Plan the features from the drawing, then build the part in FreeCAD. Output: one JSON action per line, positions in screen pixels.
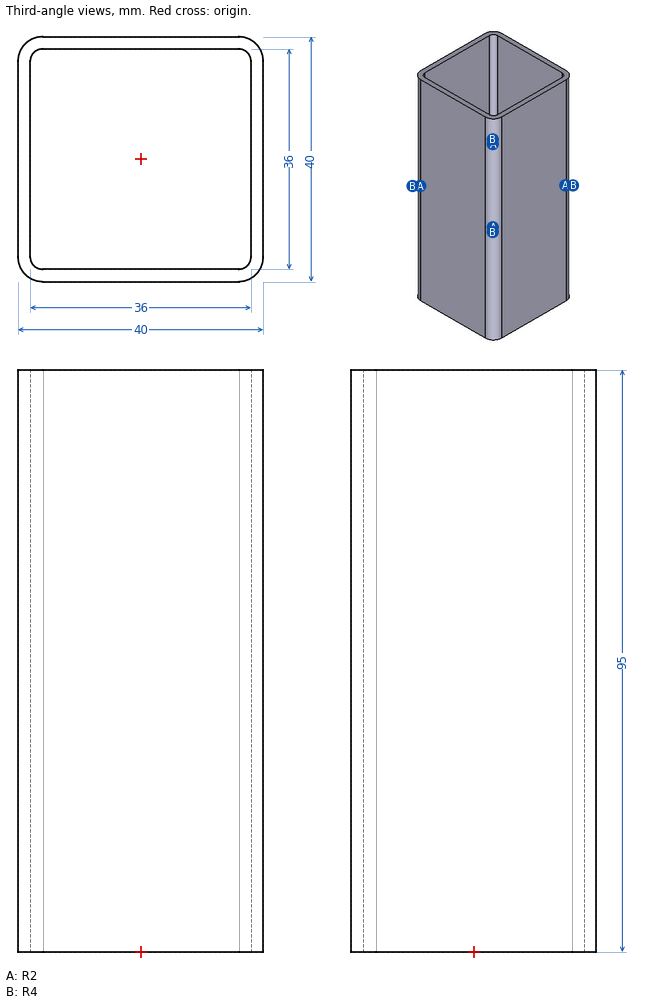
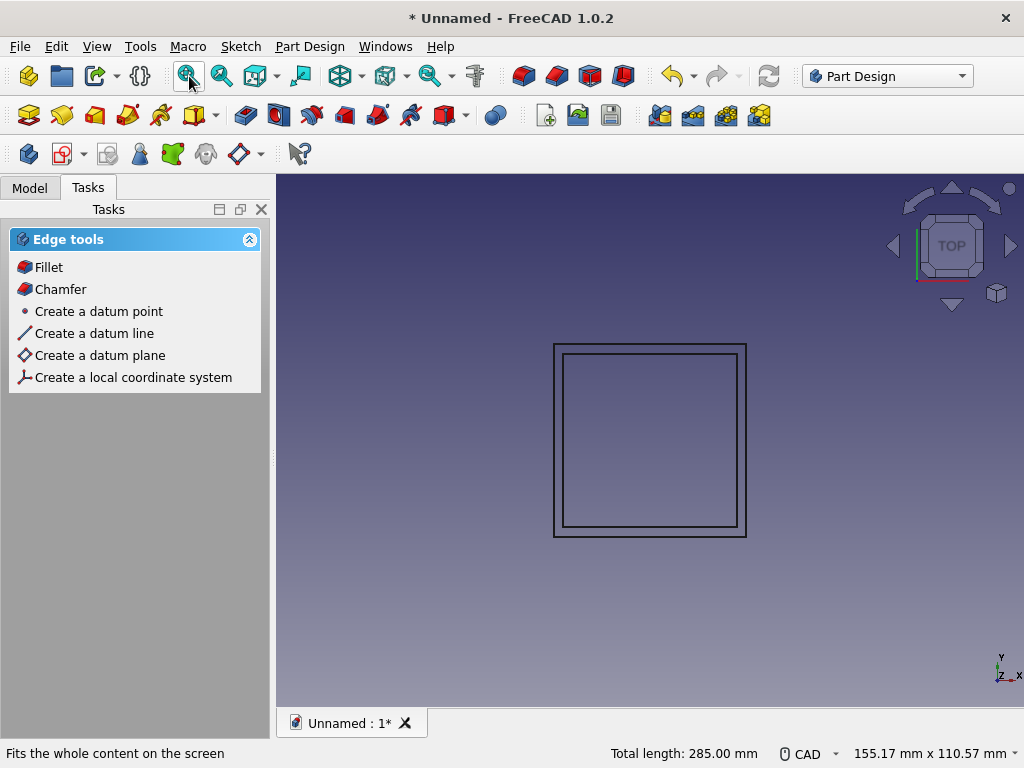
{"action": "key", "text": "v f"}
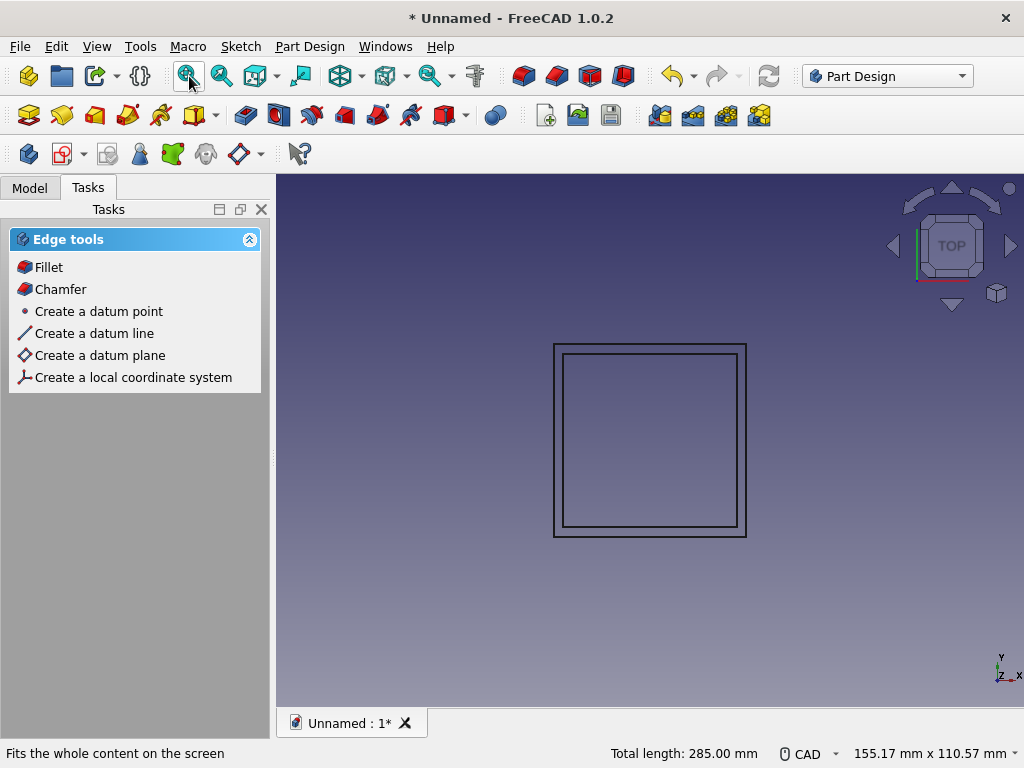
{"action": "scroll", "coordinate": [737, 526], "scroll_direction": "up", "scroll_amount": 6}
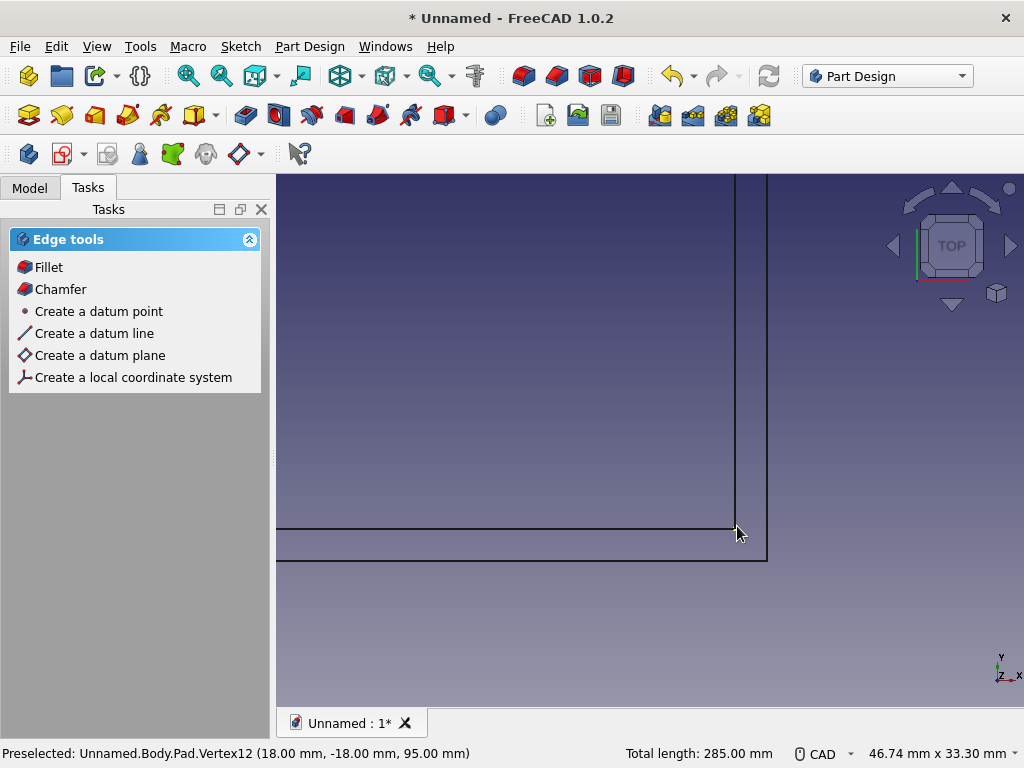
{"action": "key", "text": "v f"}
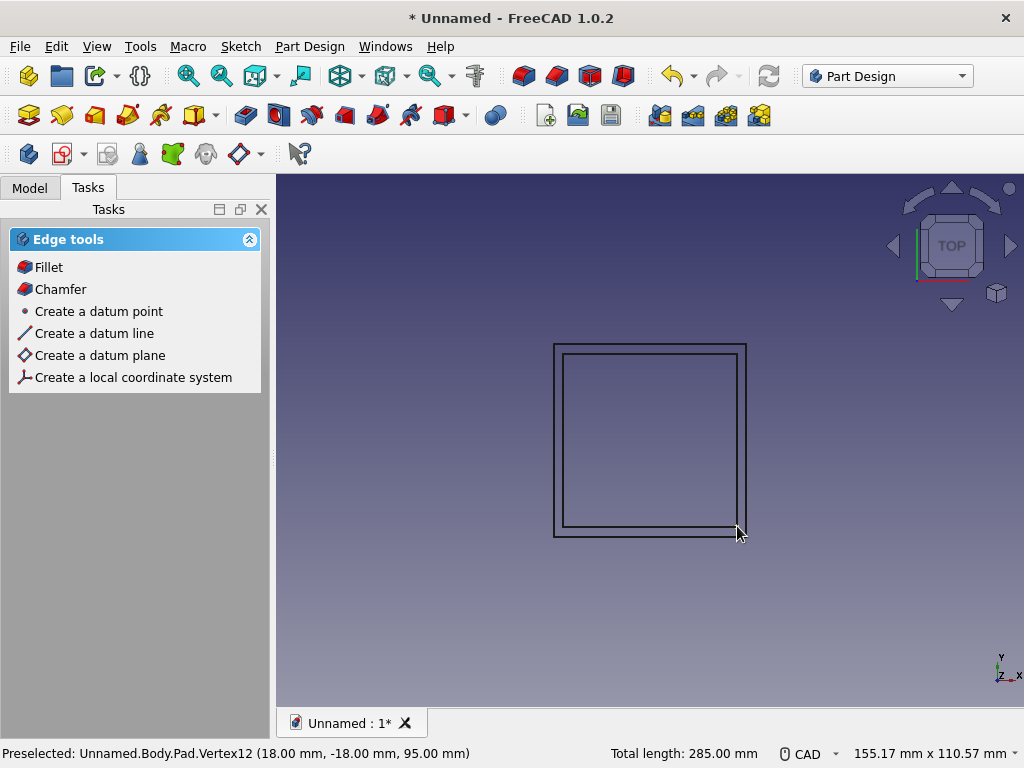
{"action": "key", "text": "1"}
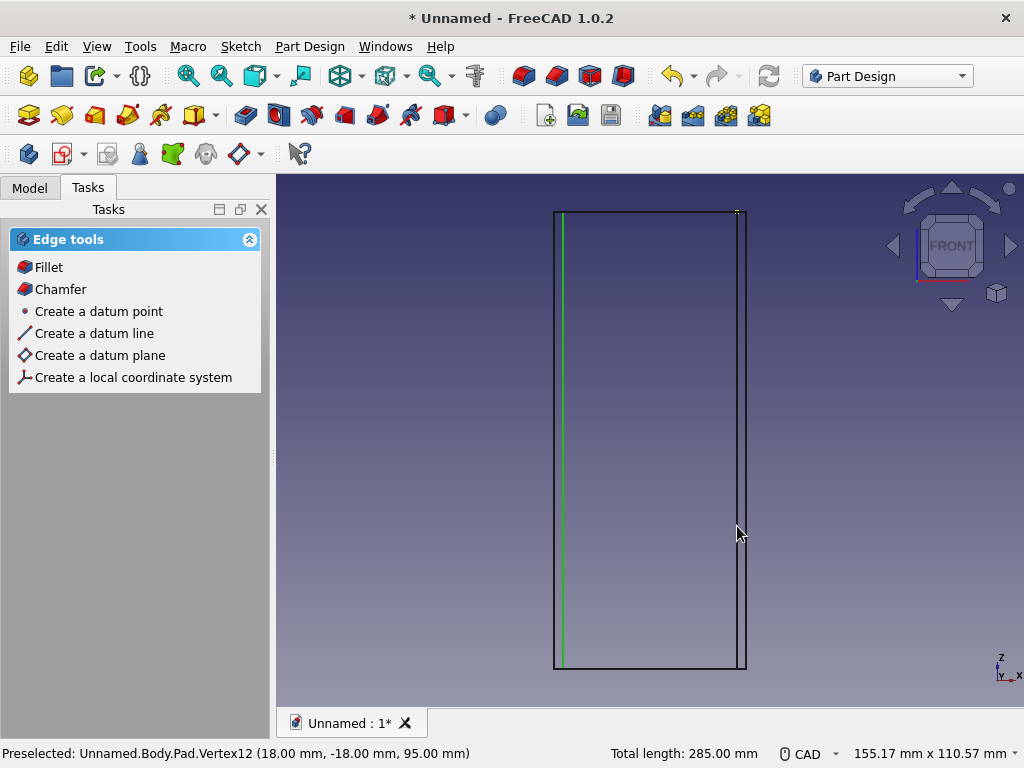
{"action": "left_click", "coordinate": [737, 439], "text": "ctrl"}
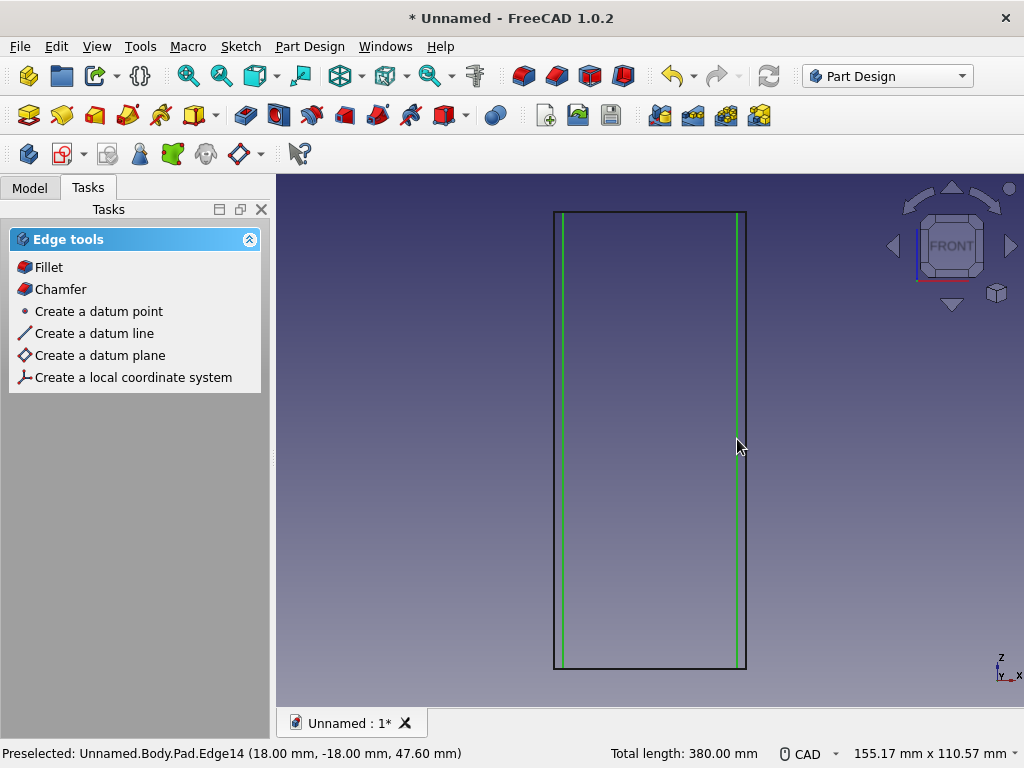
{"action": "key", "text": "v 1"}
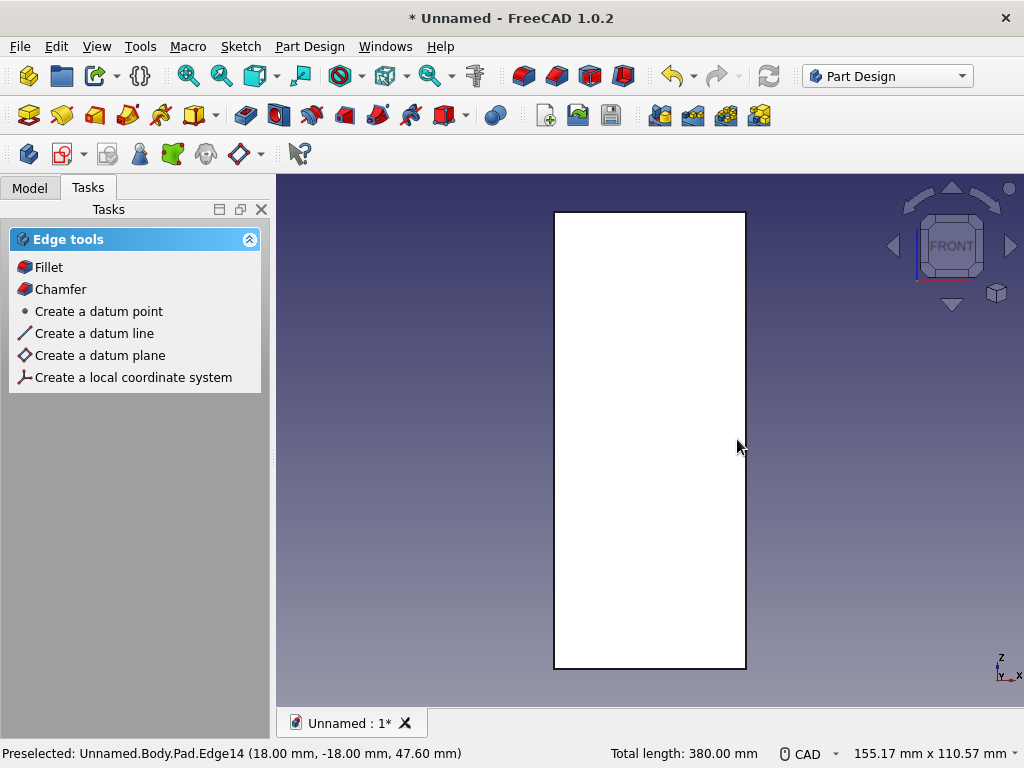
{"action": "left_click", "coordinate": [524, 76]}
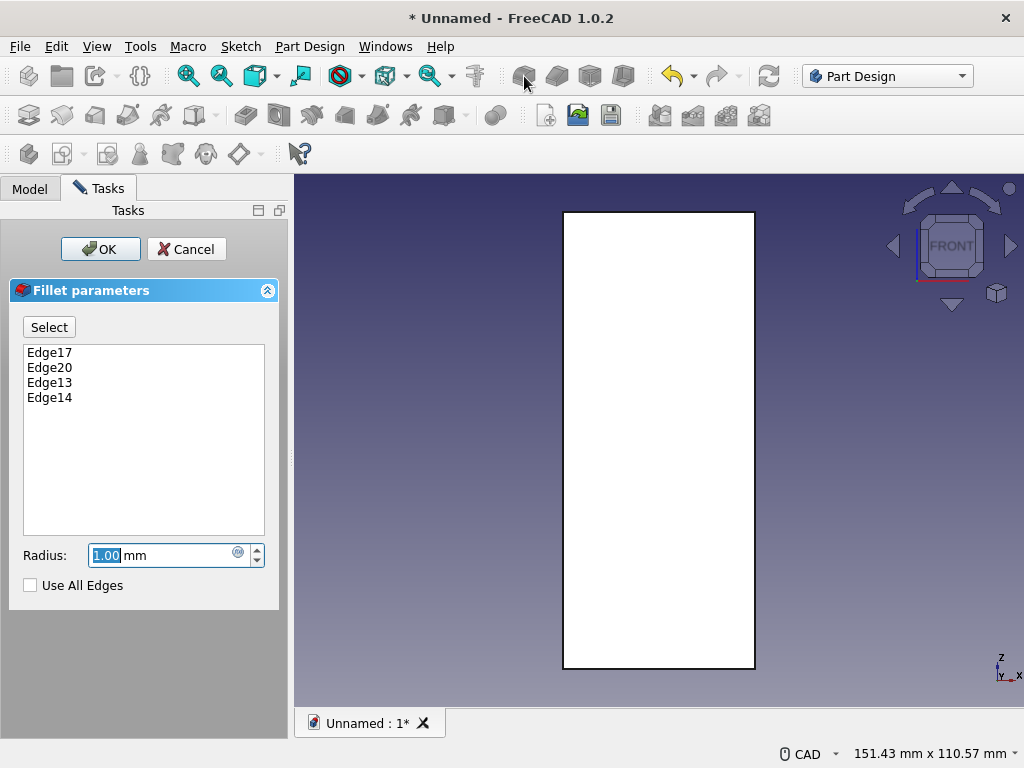
{"action": "type", "text": "2"}
{"action": "key", "text": "Tab"}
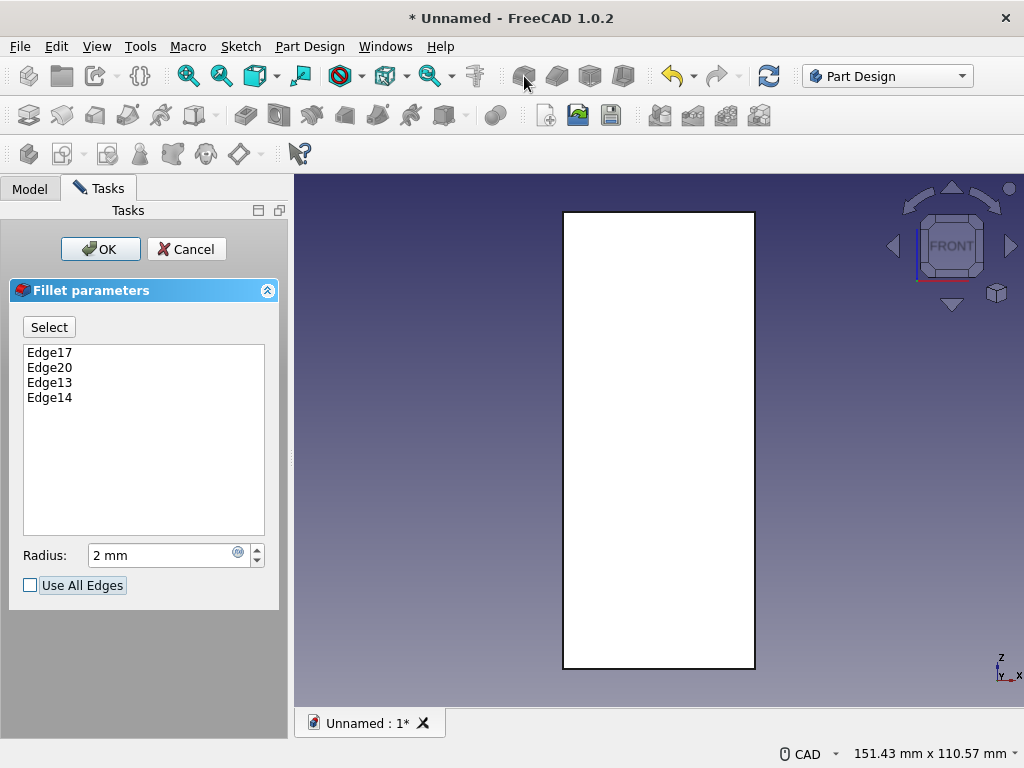
{"action": "left_click", "coordinate": [101, 249]}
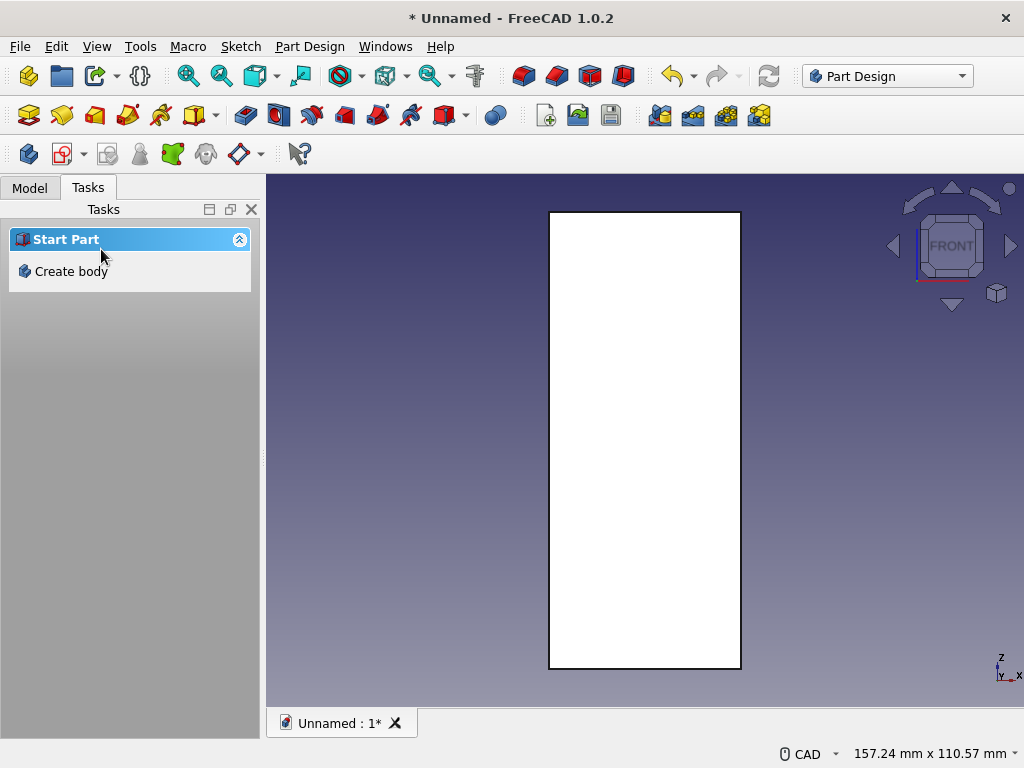
{"action": "left_click", "coordinate": [741, 439]}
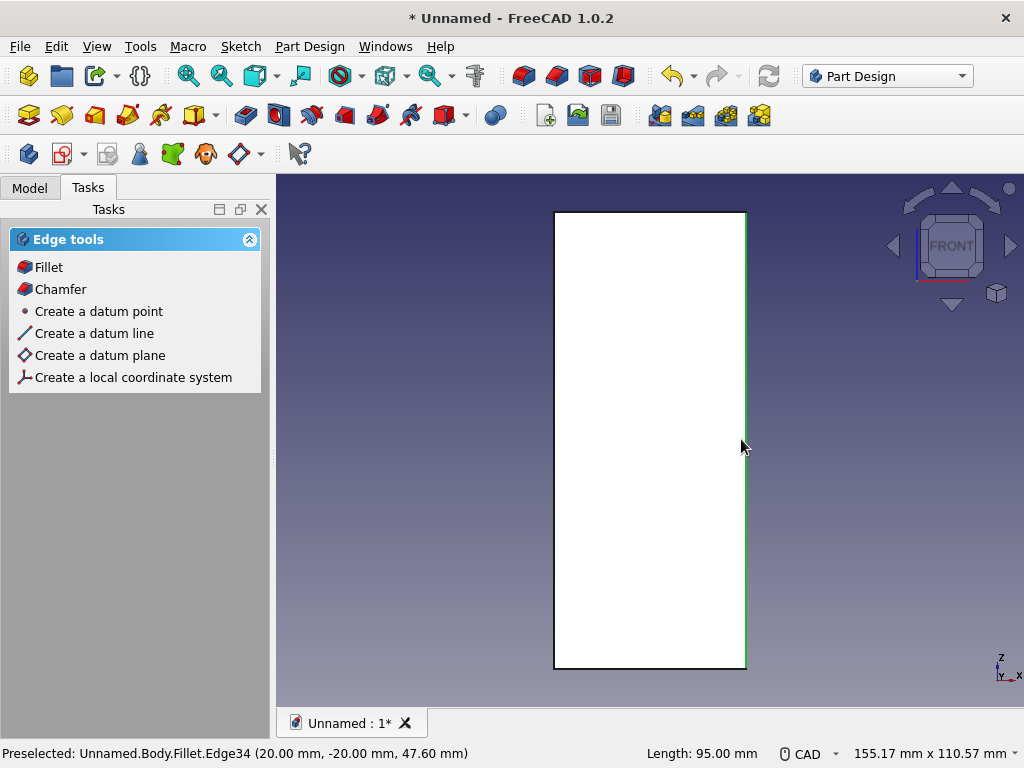
{"action": "left_click", "coordinate": [554, 439], "text": "ctrl"}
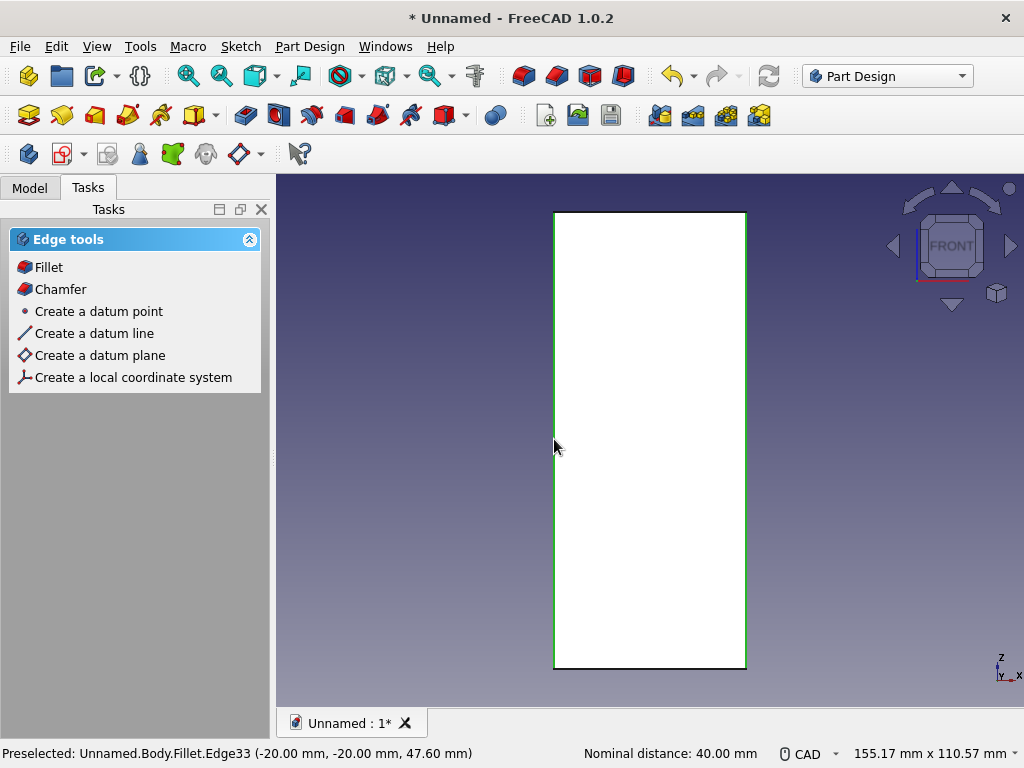
{"action": "key", "text": "0"}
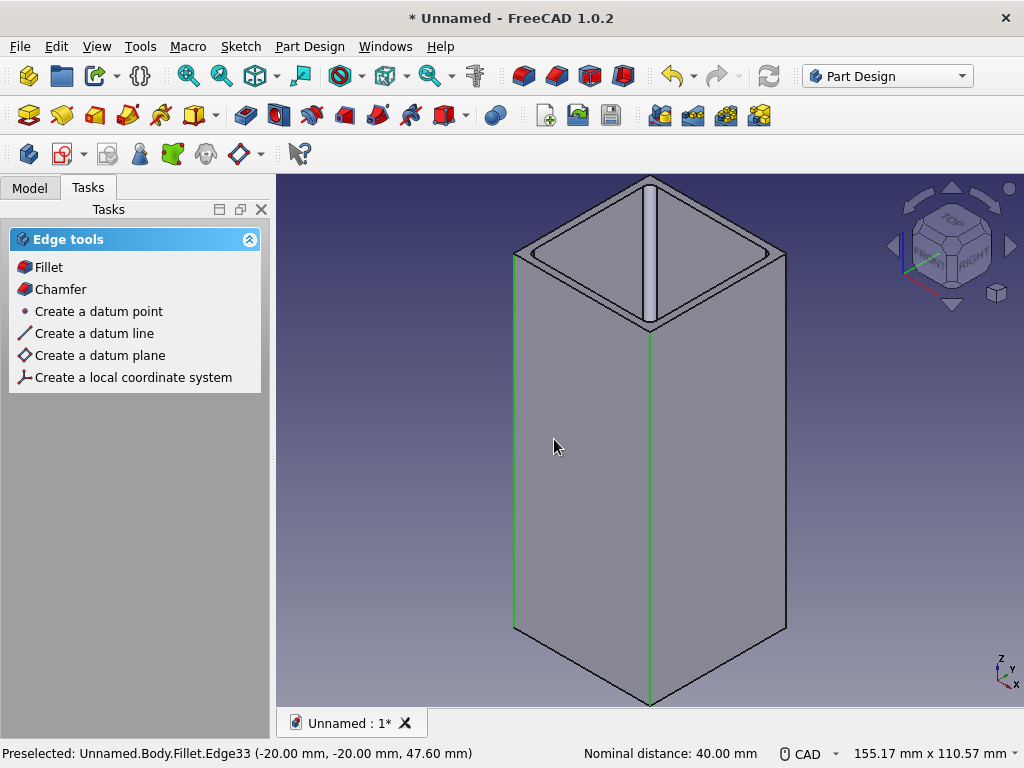
{"action": "key", "text": "2"}